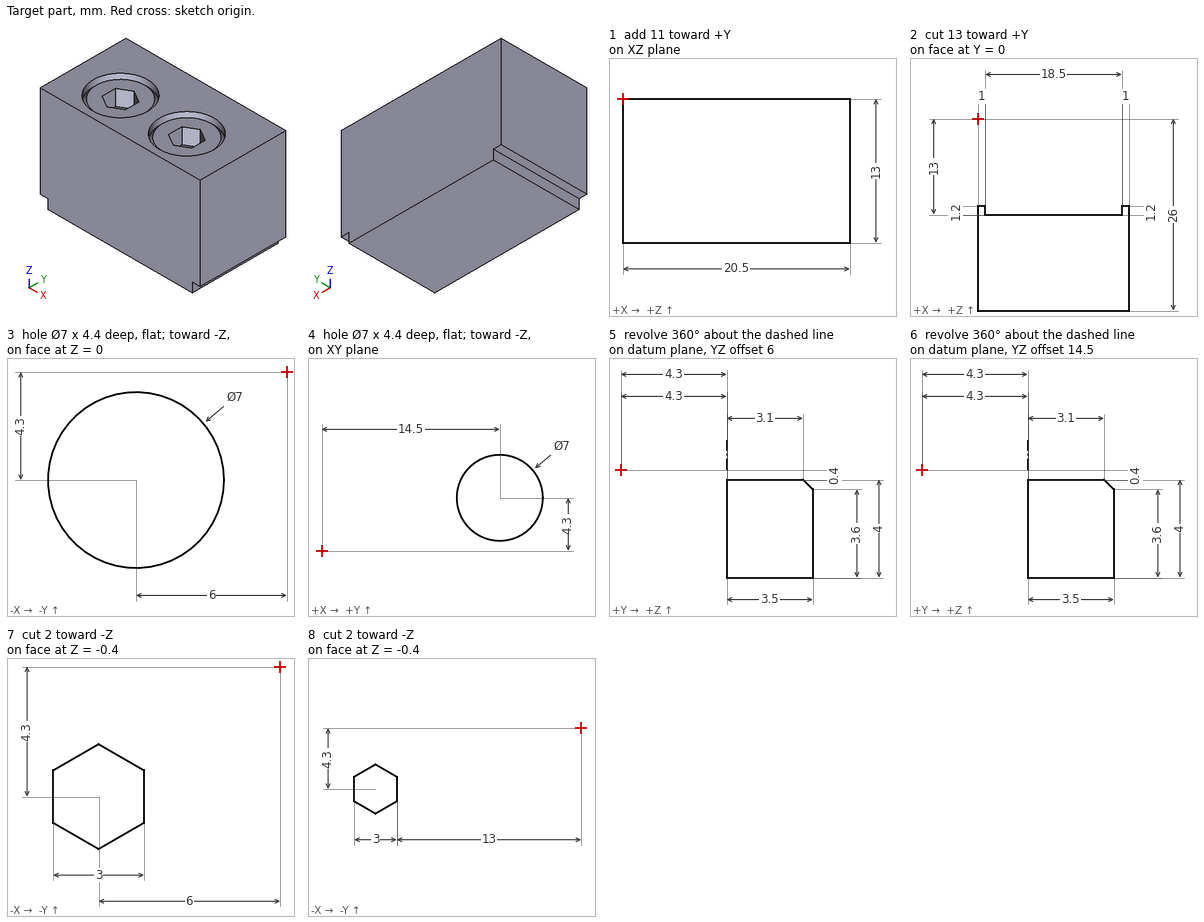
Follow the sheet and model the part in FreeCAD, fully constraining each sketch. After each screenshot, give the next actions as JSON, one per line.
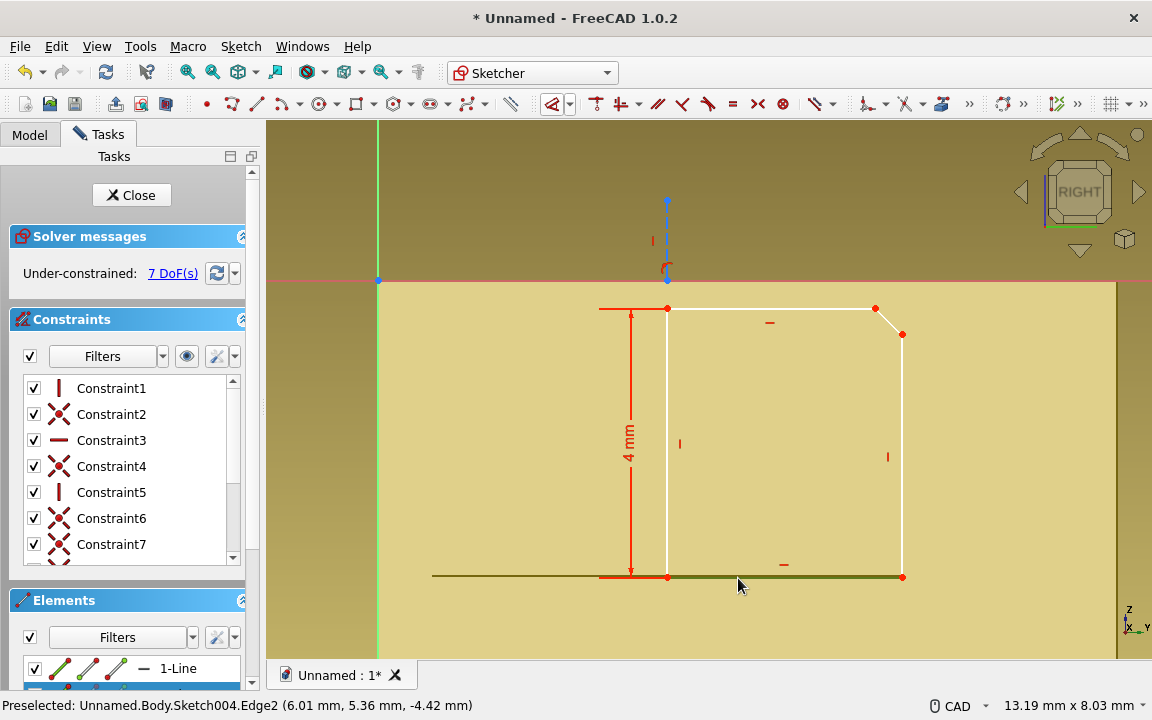
{"action": "left_click", "coordinate": [570, 104]}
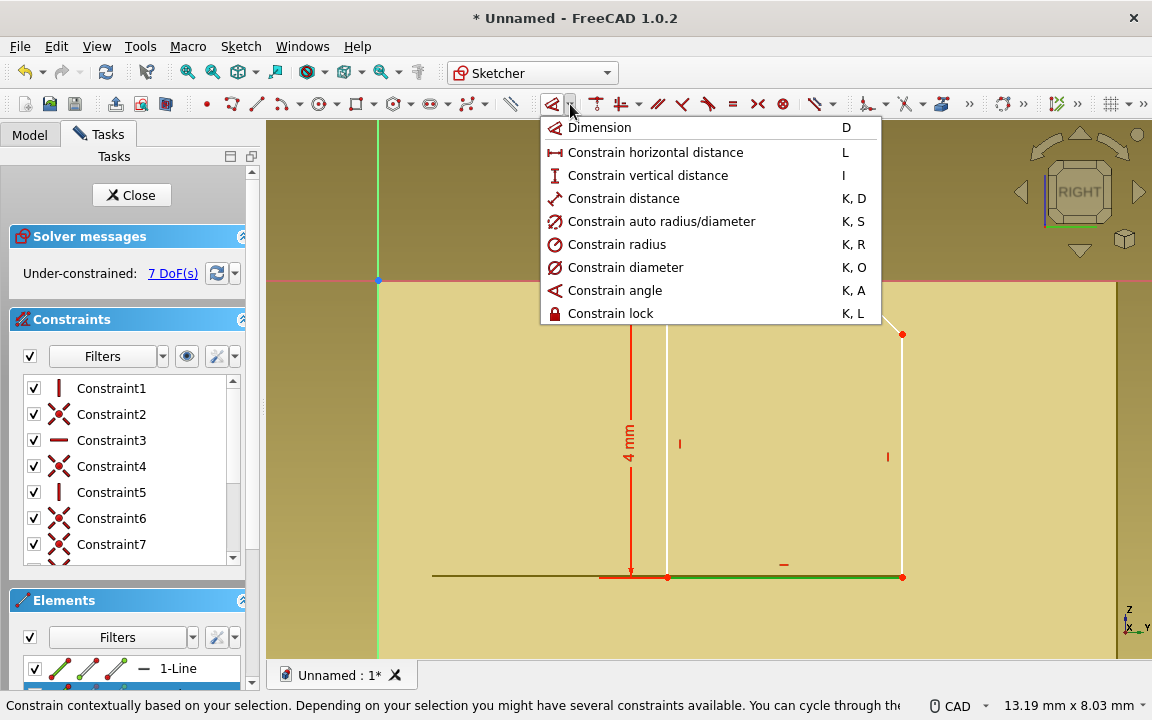
{"action": "left_click", "coordinate": [711, 152]}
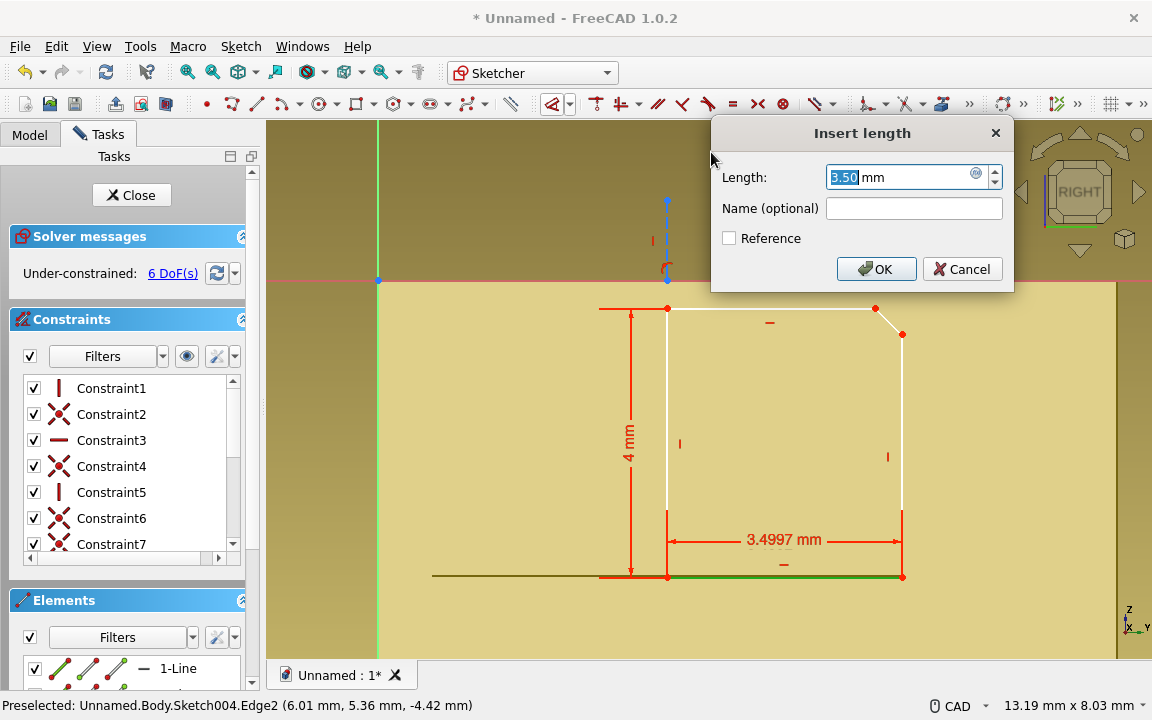
{"action": "type", "text": "3.5"}
{"action": "key", "text": "Return"}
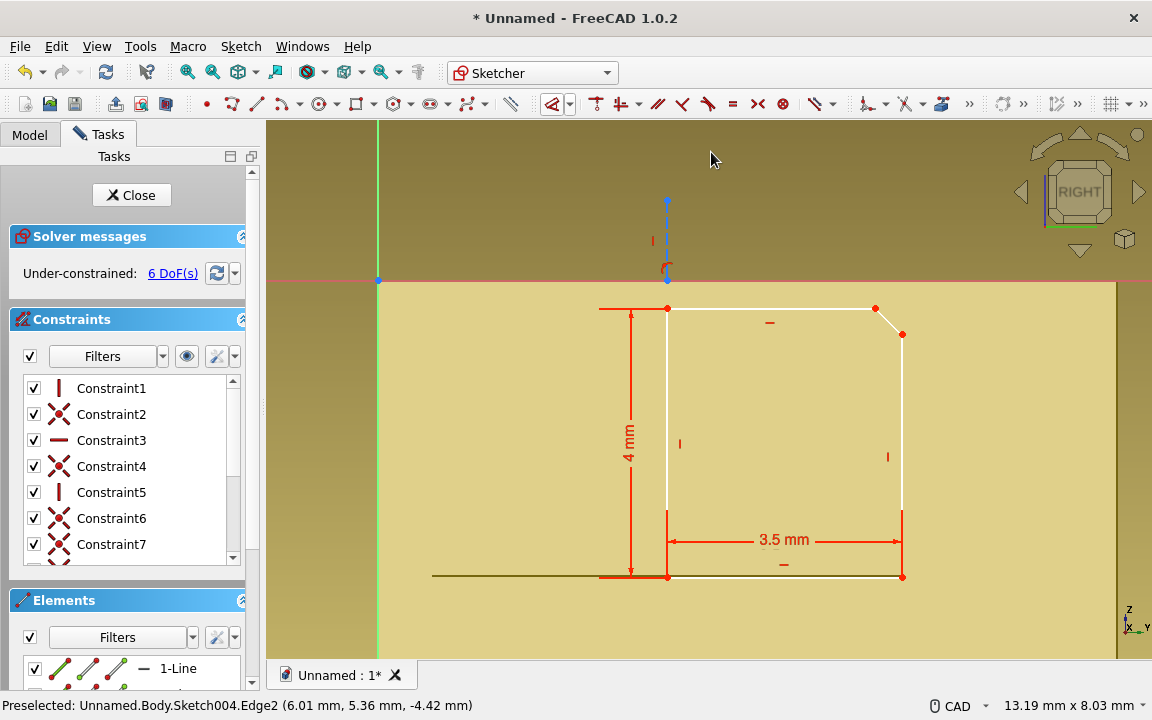
{"action": "left_click", "coordinate": [902, 505]}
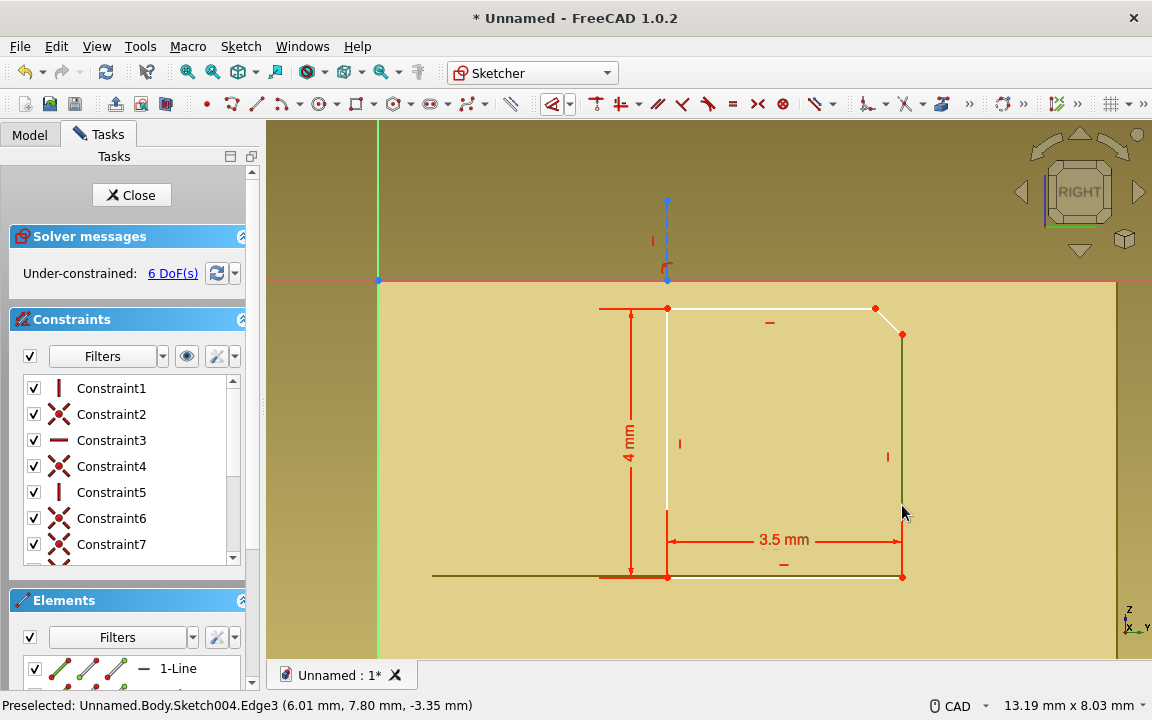
{"action": "key", "text": "i"}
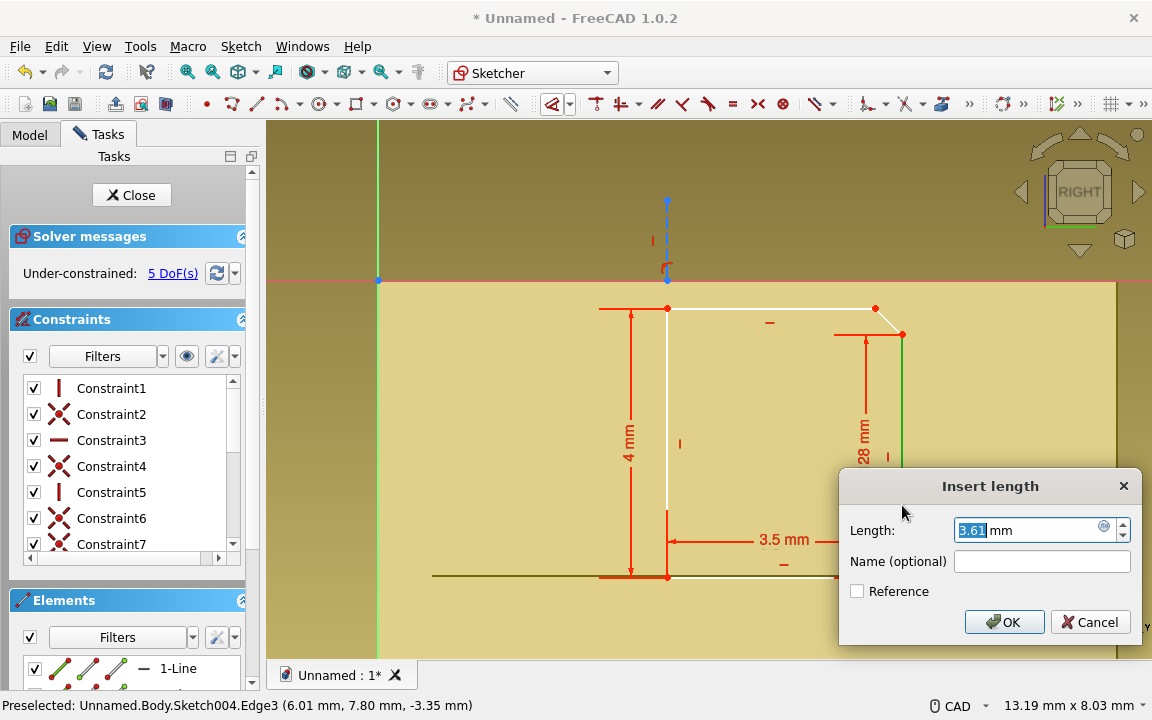
{"action": "type", "text": "3.6"}
{"action": "key", "text": "Return"}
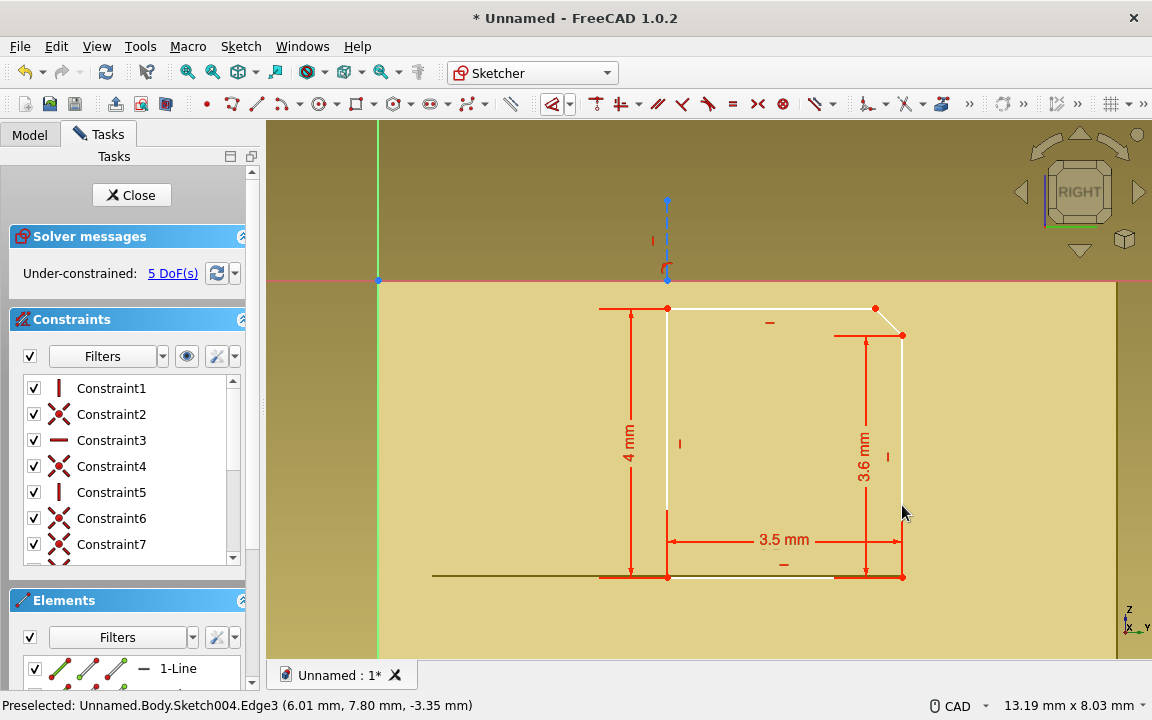
{"action": "left_click", "coordinate": [813, 309]}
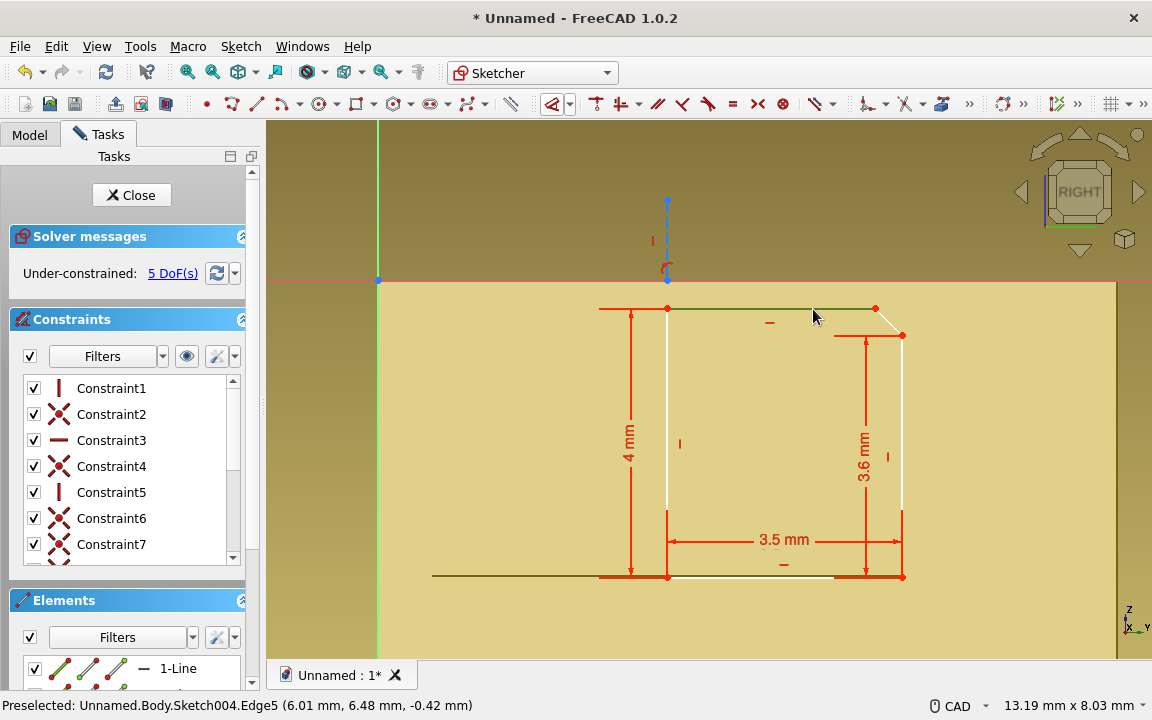
{"action": "key", "text": "l"}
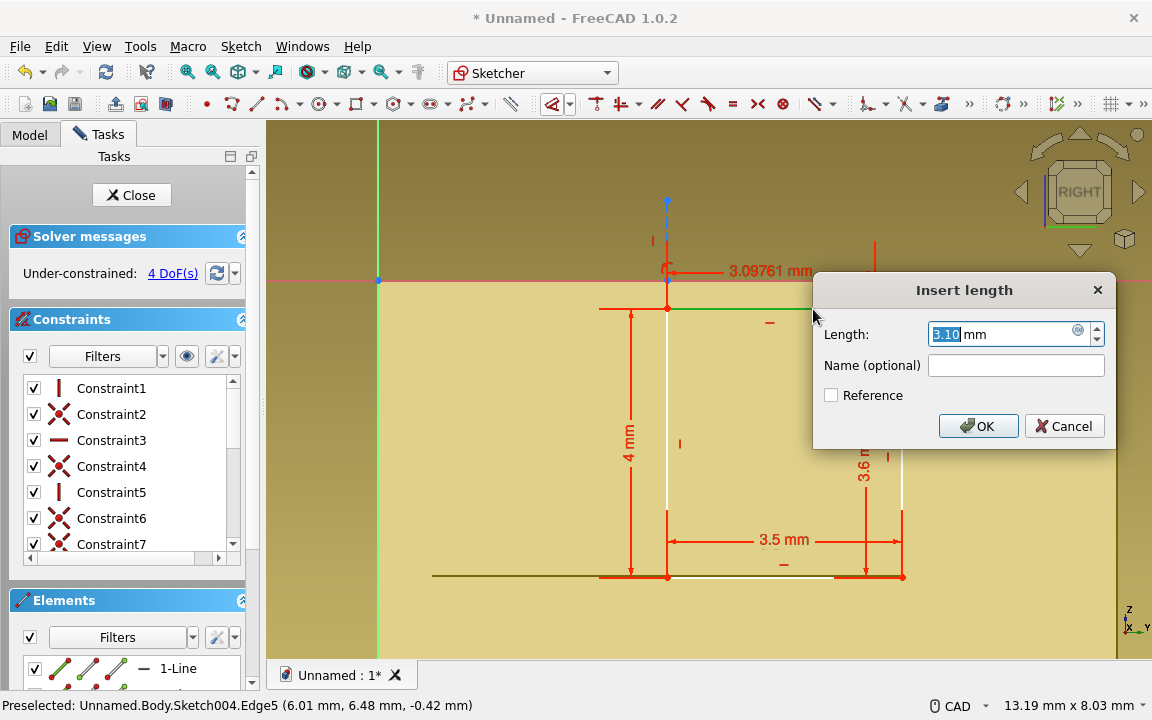
{"action": "type", "text": "3.1"}
{"action": "key", "text": "Return"}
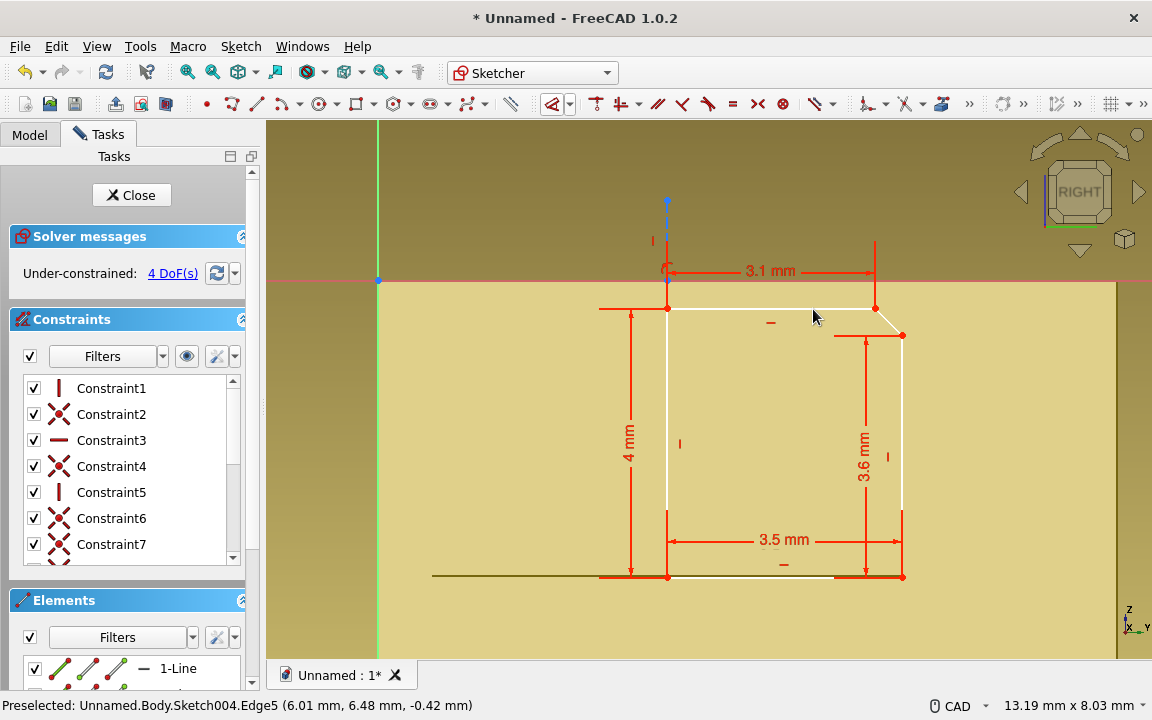
{"action": "left_click", "coordinate": [667, 309]}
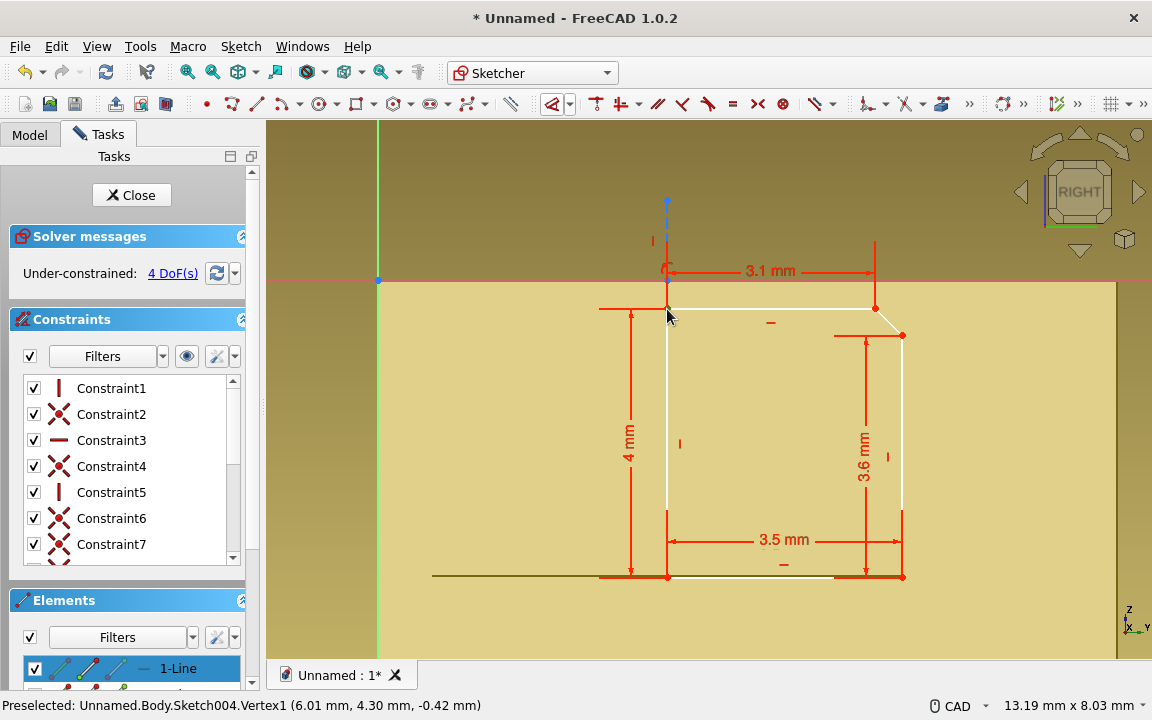
{"action": "left_click", "coordinate": [570, 104]}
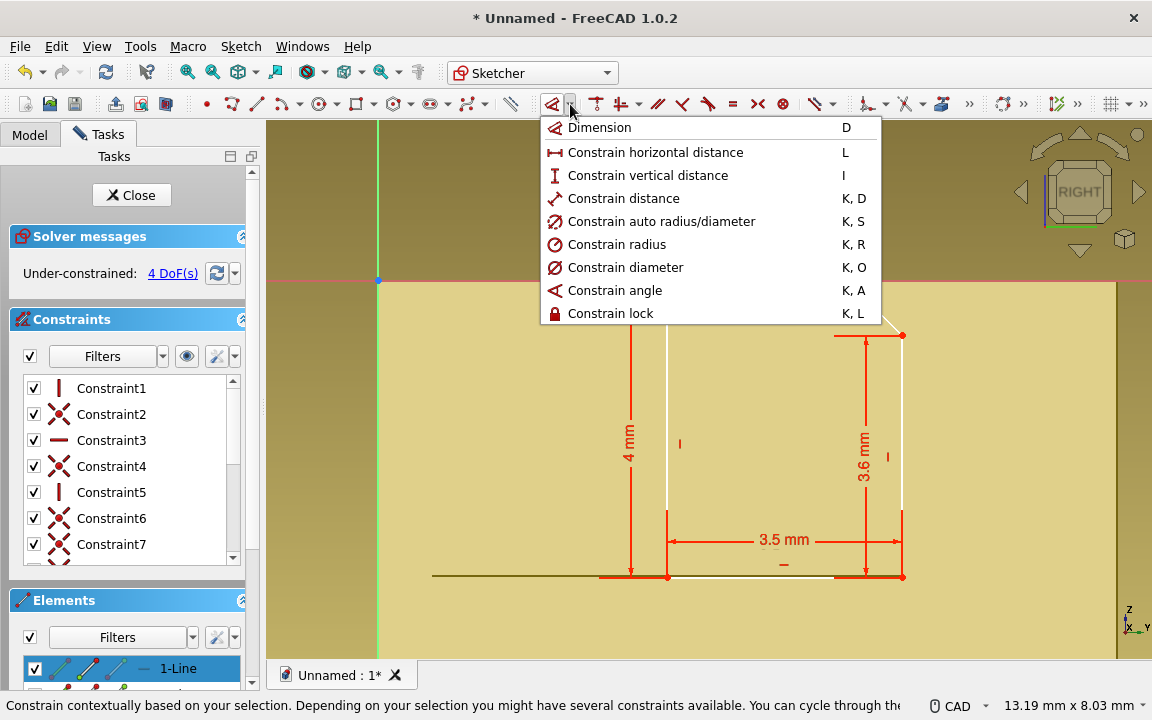
{"action": "left_click", "coordinate": [711, 152]}